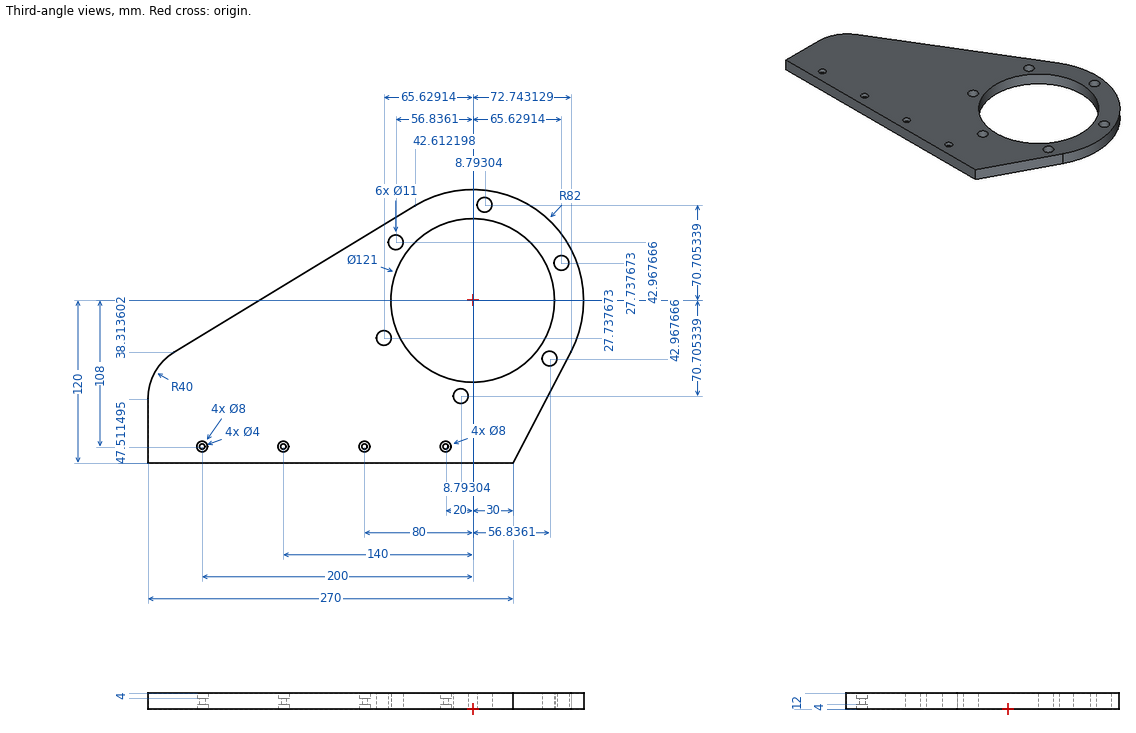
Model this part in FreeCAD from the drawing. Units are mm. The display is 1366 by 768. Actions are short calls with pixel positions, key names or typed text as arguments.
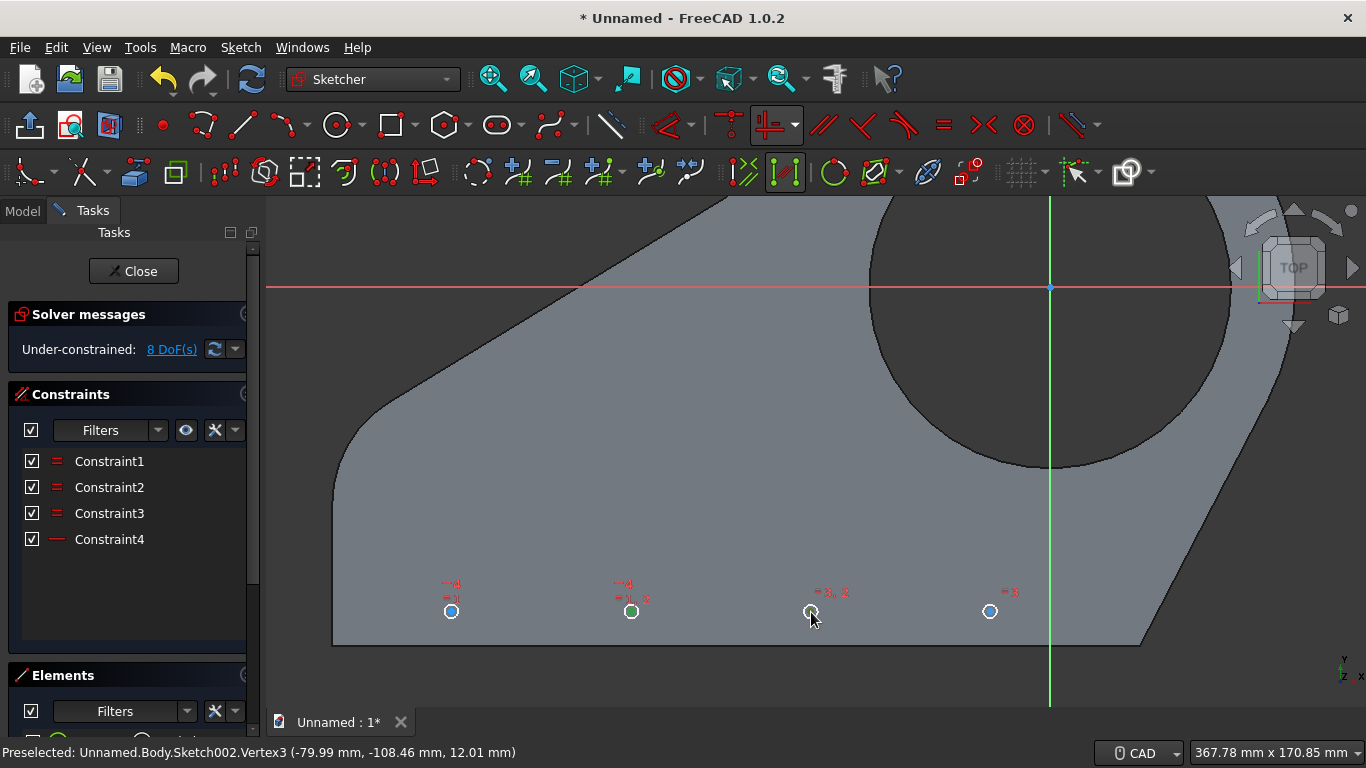
click(798, 126)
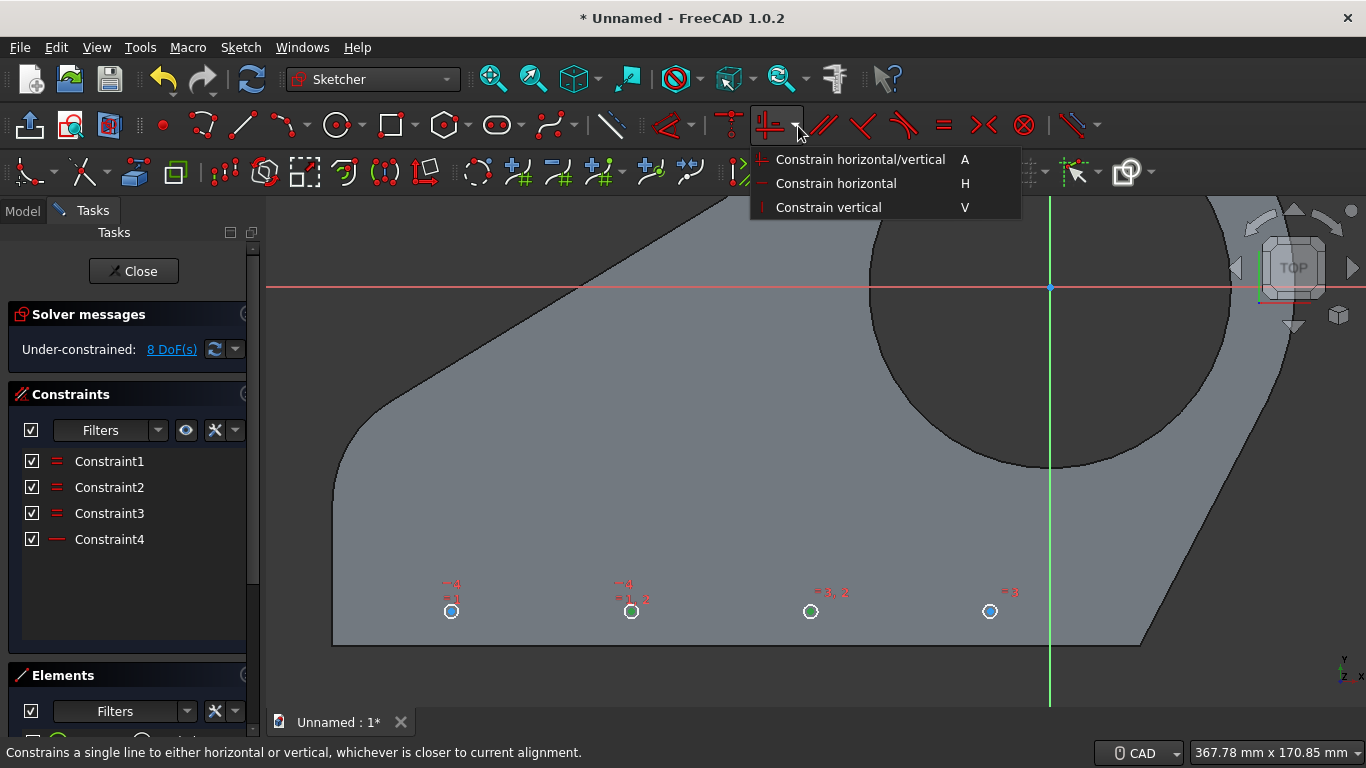
click(886, 183)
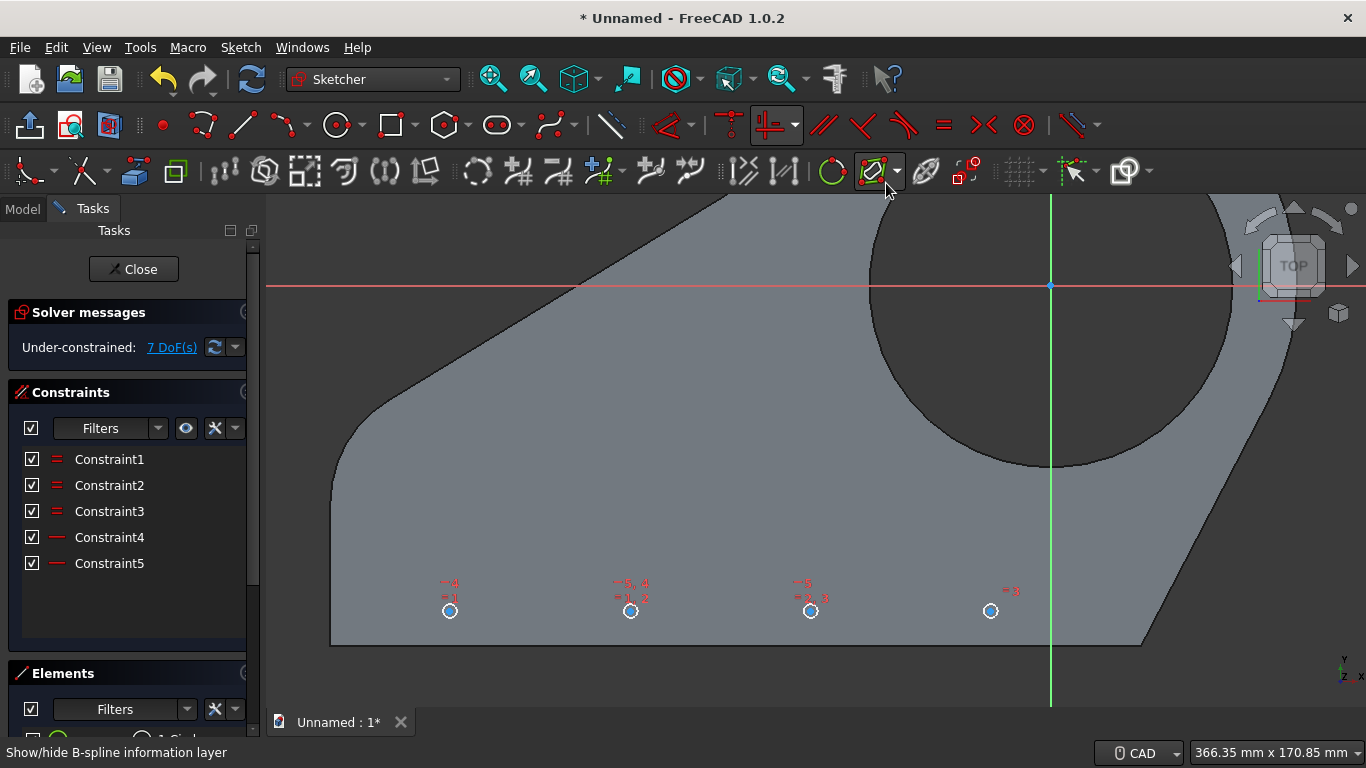
click(811, 611)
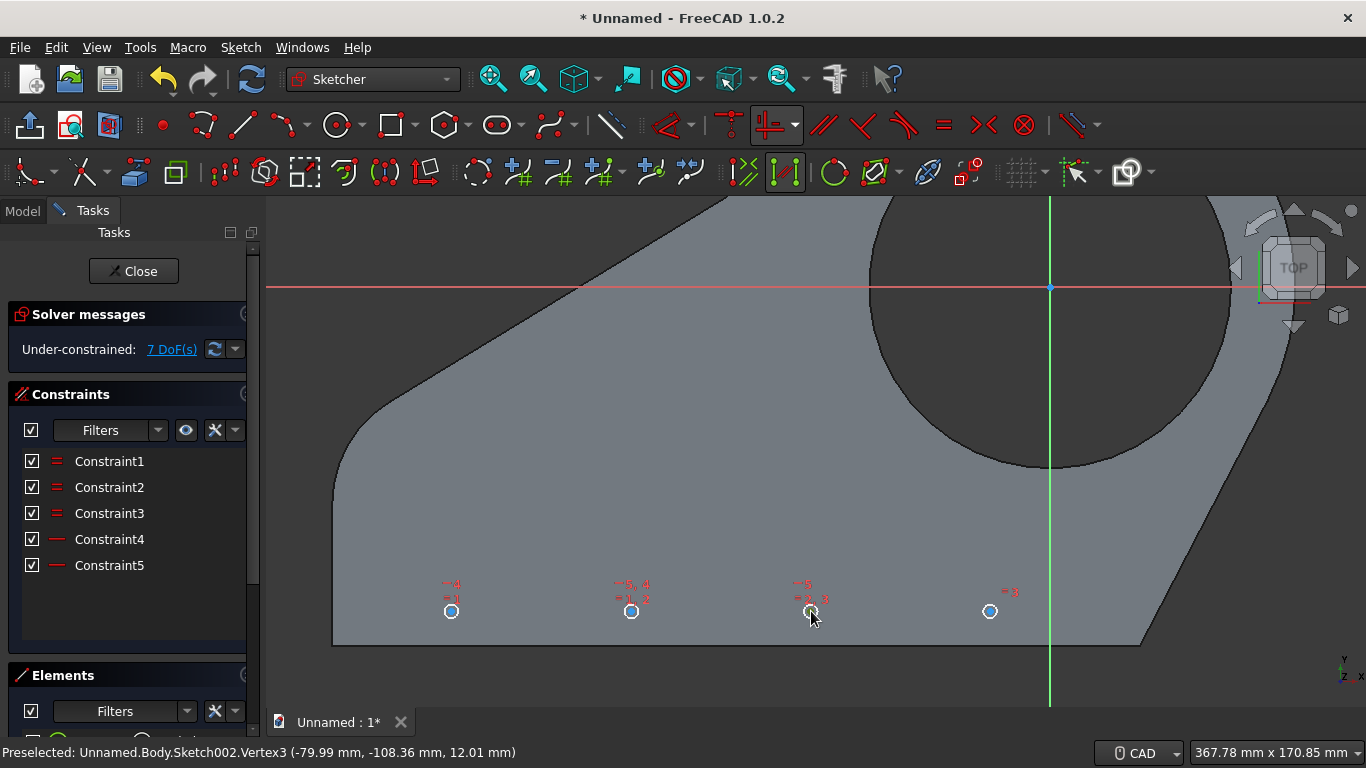
click(990, 611)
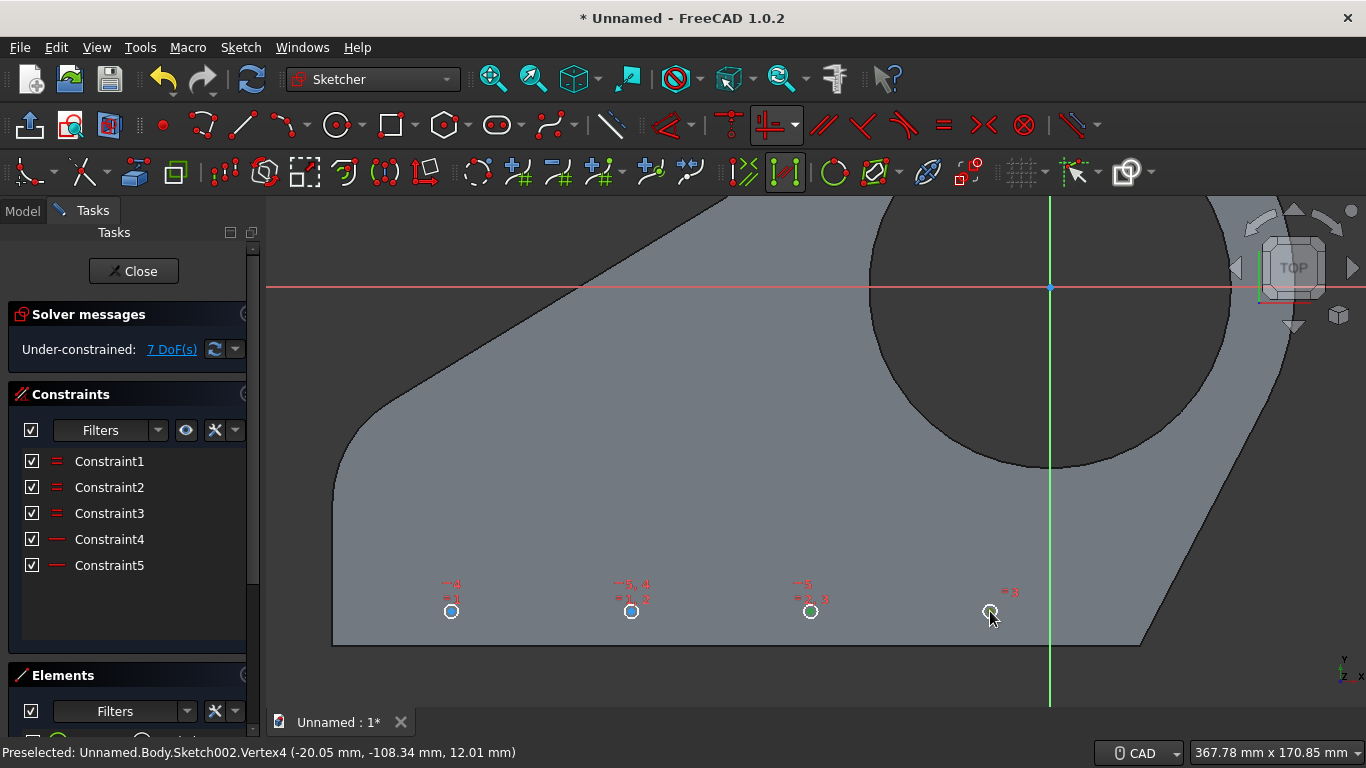
click(798, 126)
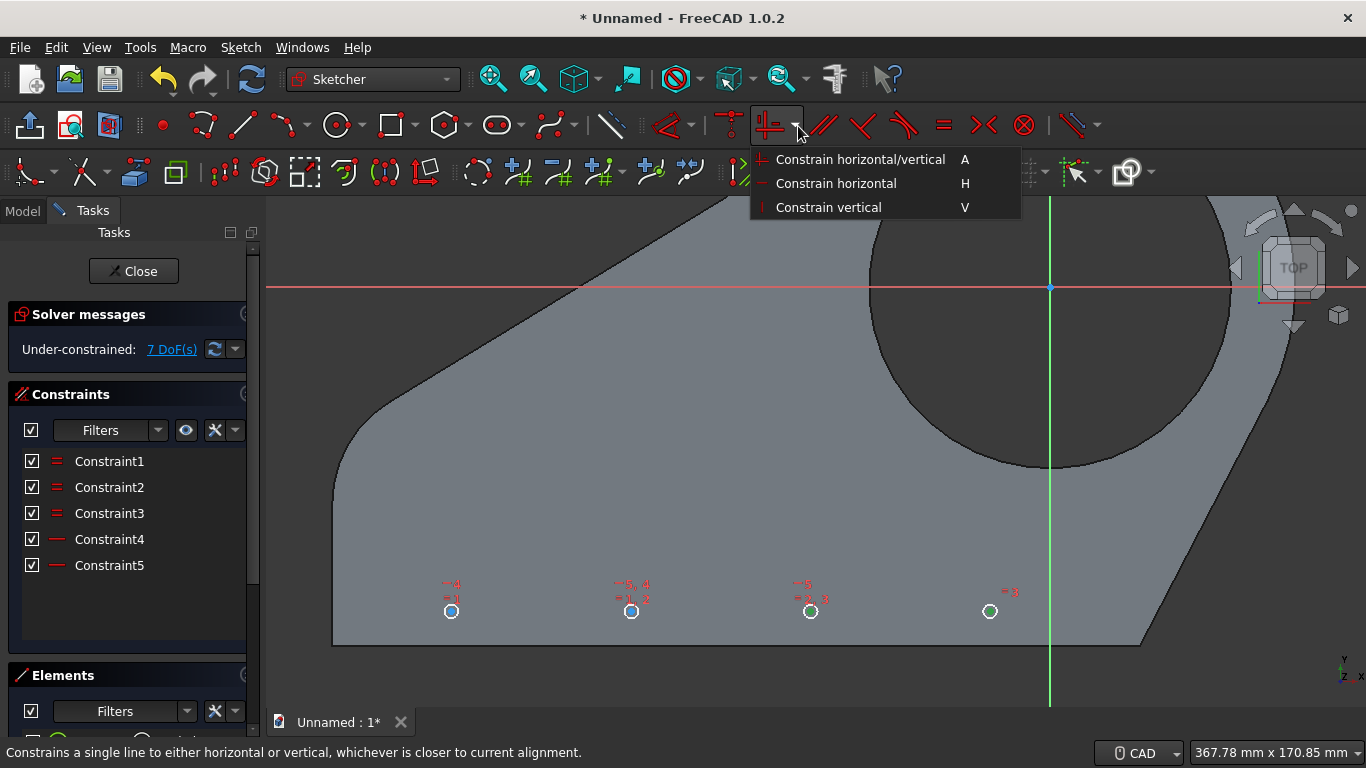
click(886, 183)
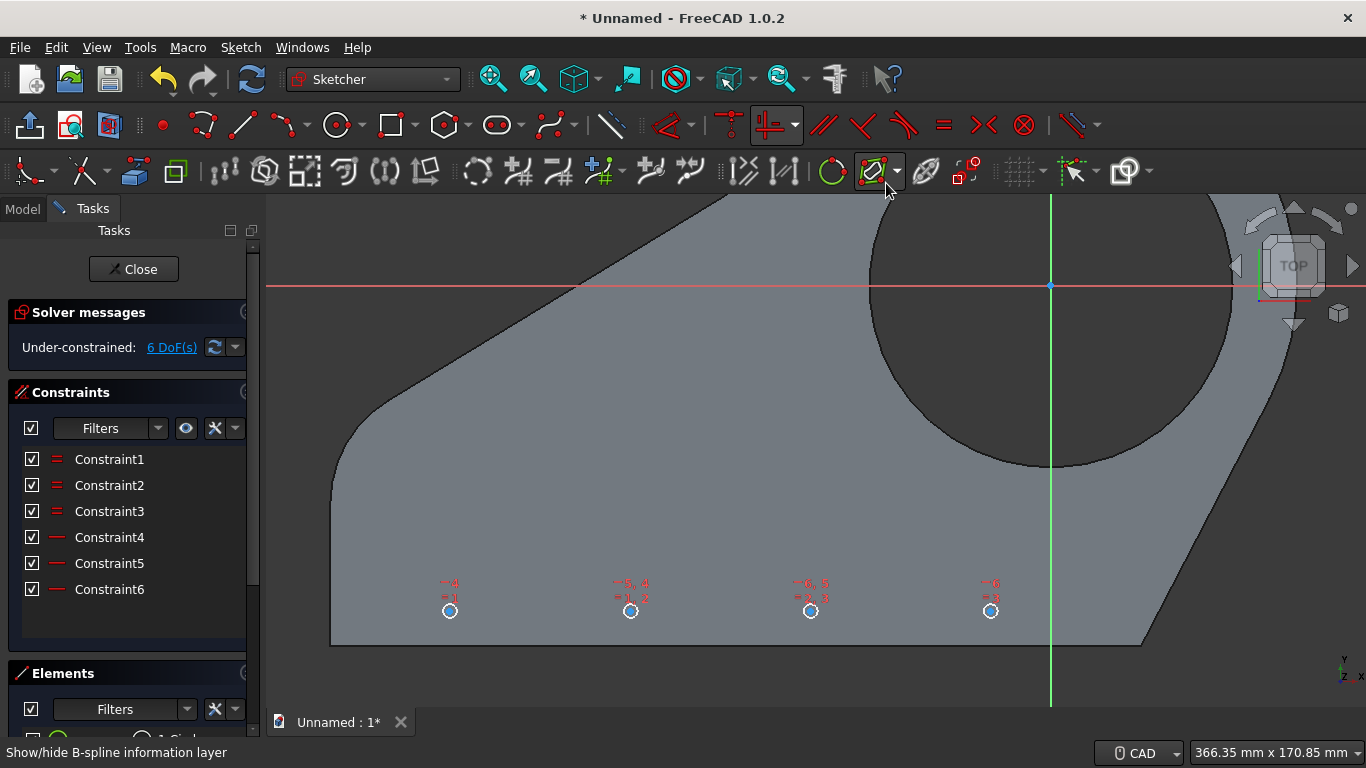
click(666, 126)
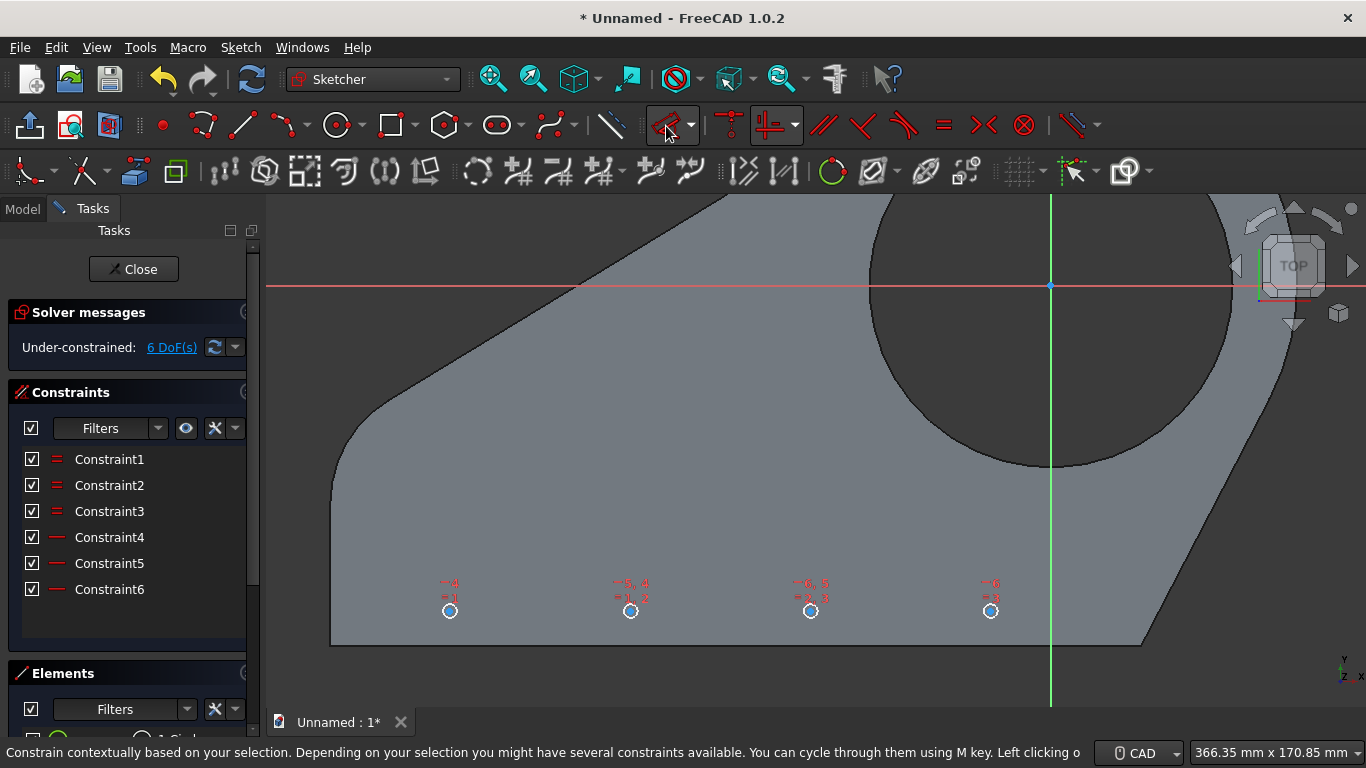
scroll(450, 604, up, 6)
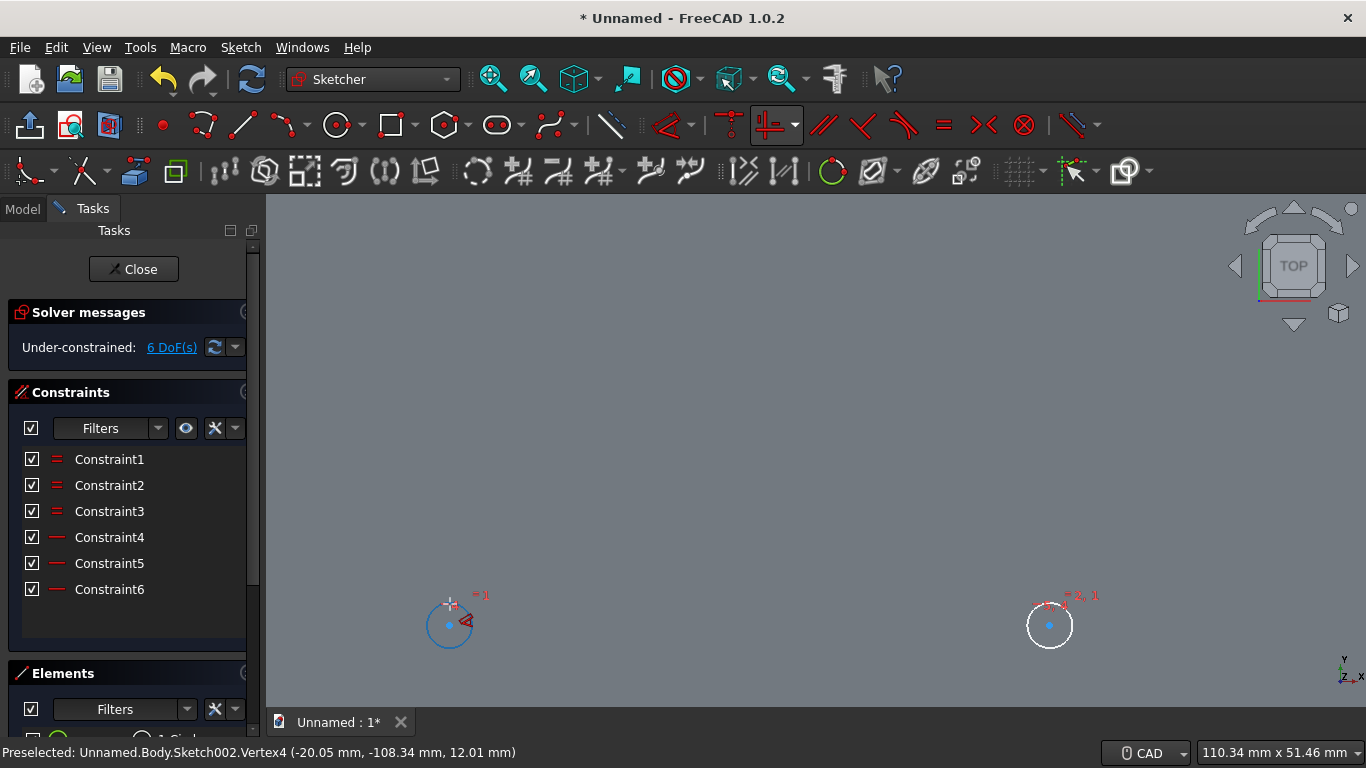
click(450, 603)
click(451, 571)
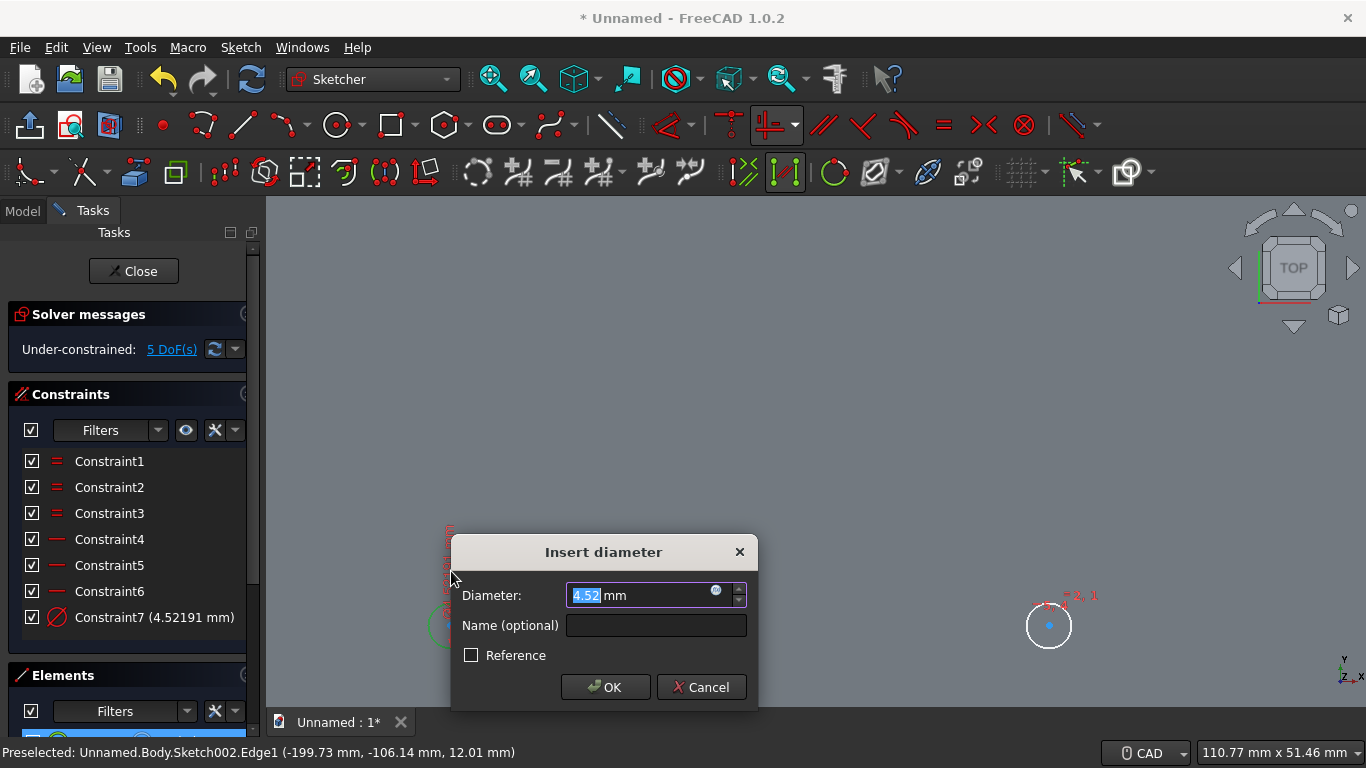
text(4)
key(Return)